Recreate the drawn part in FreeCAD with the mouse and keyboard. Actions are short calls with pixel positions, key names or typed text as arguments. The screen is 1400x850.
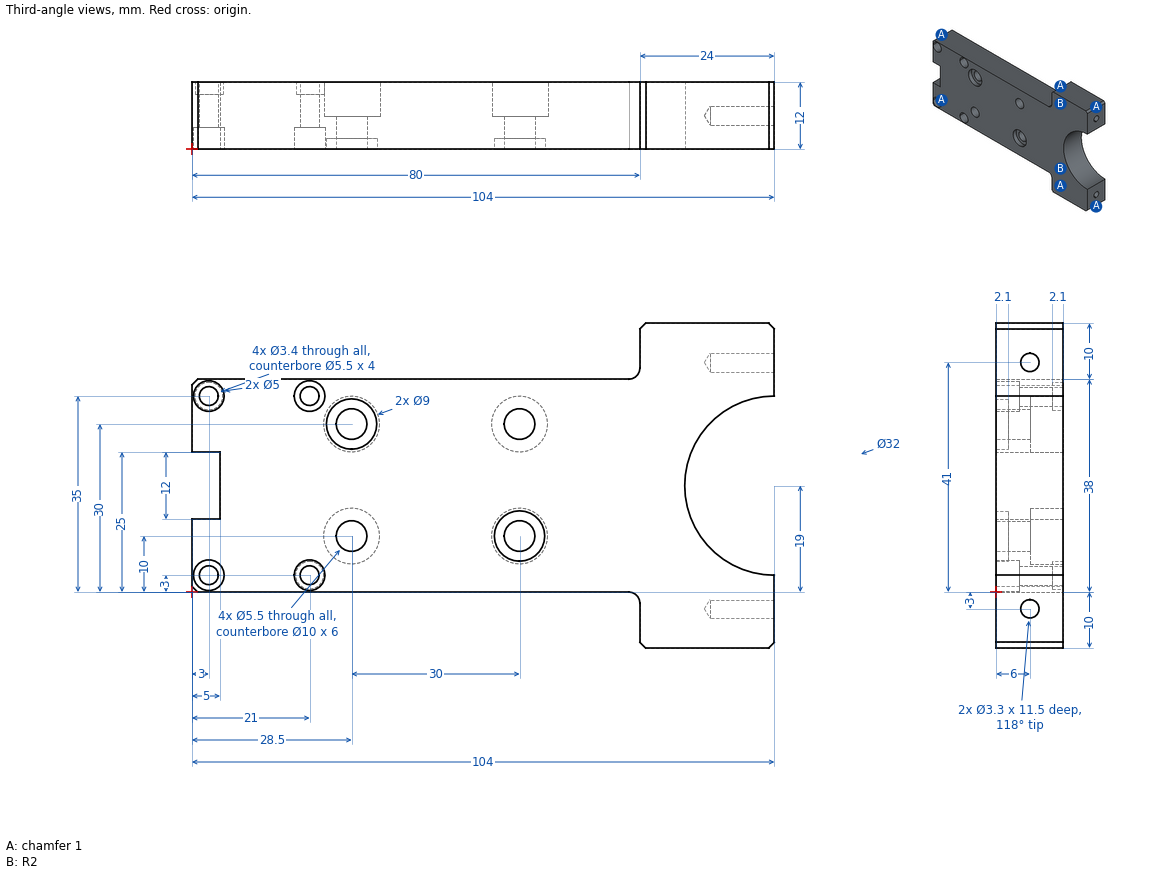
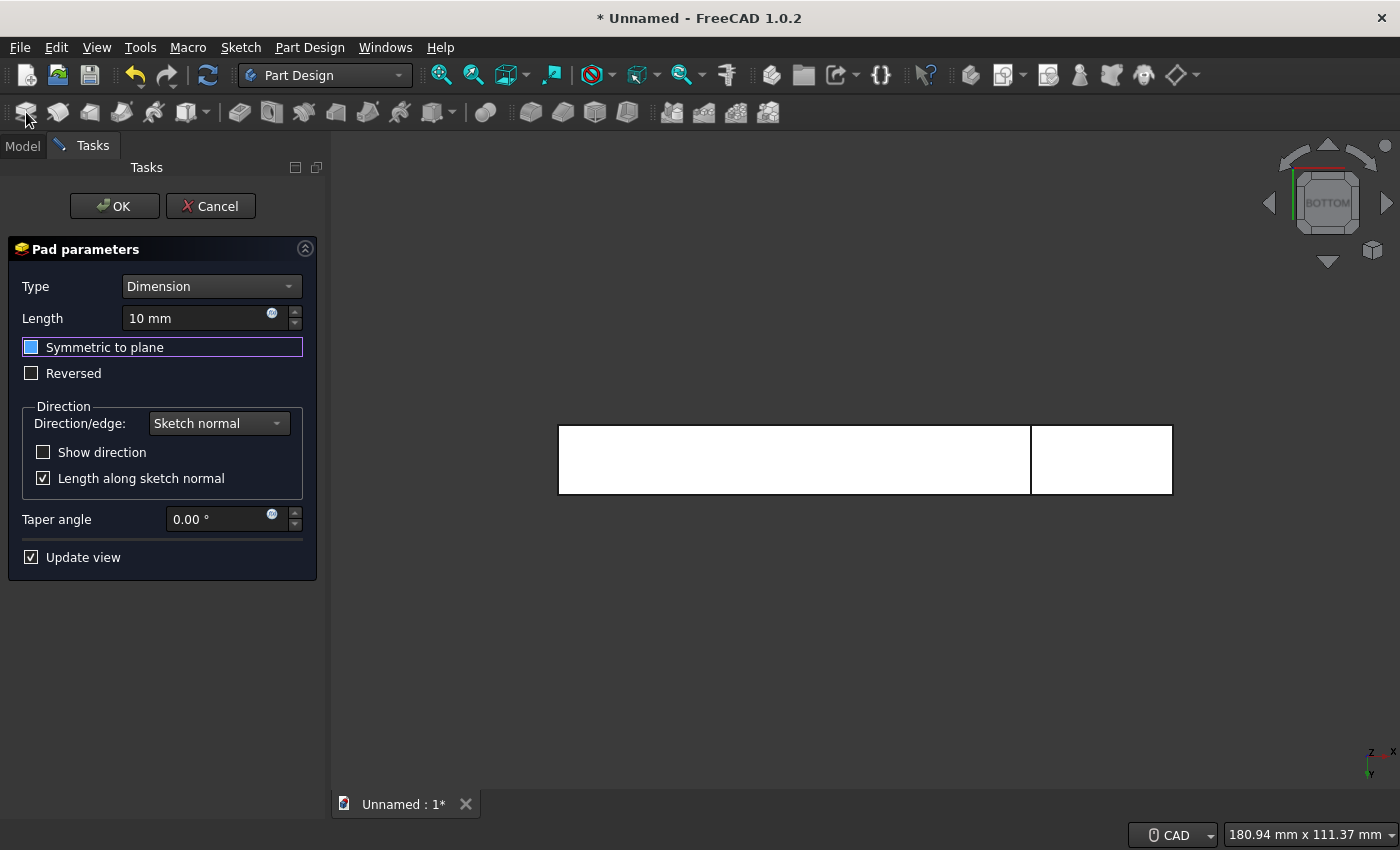
click(115, 206)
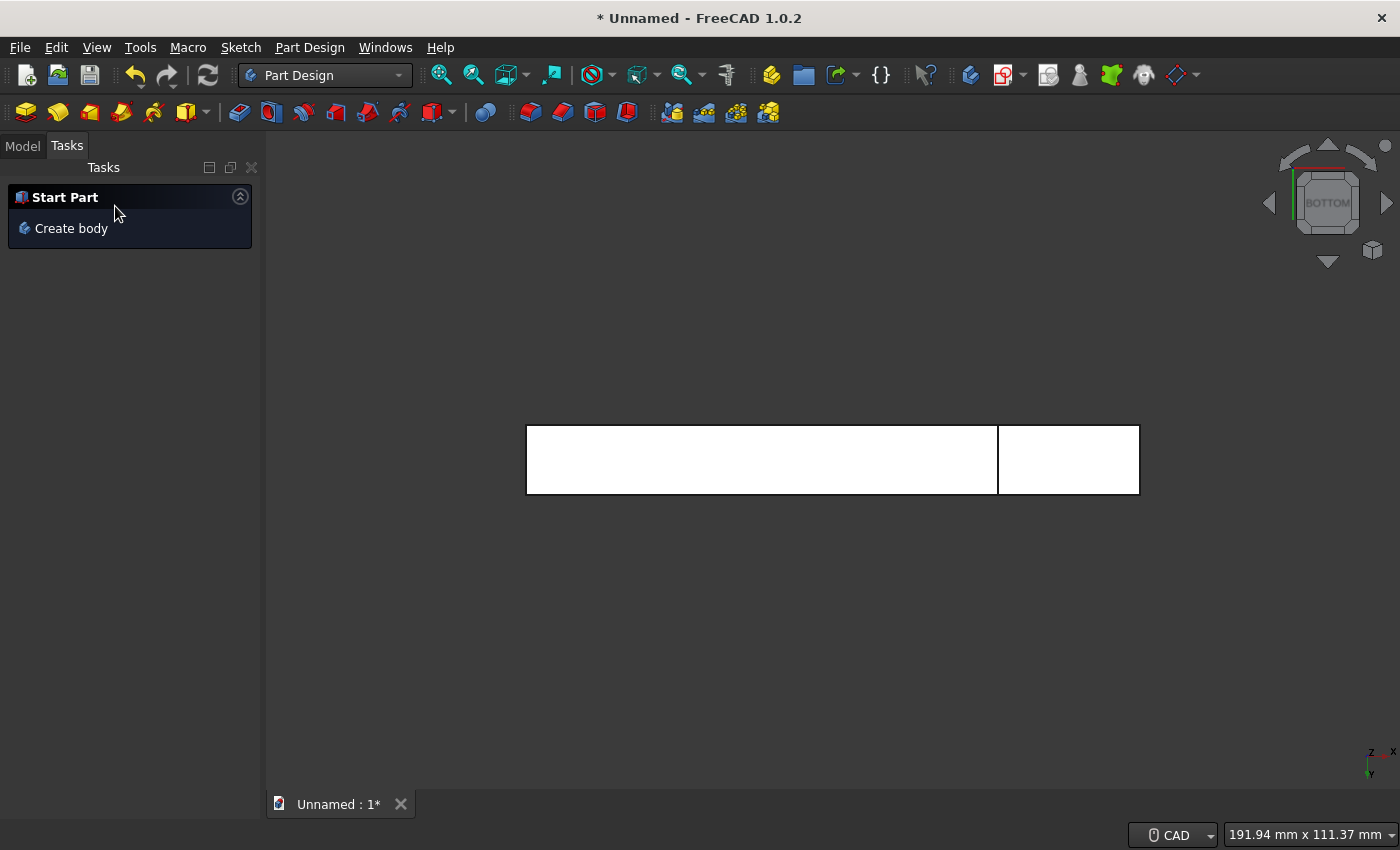
key(0)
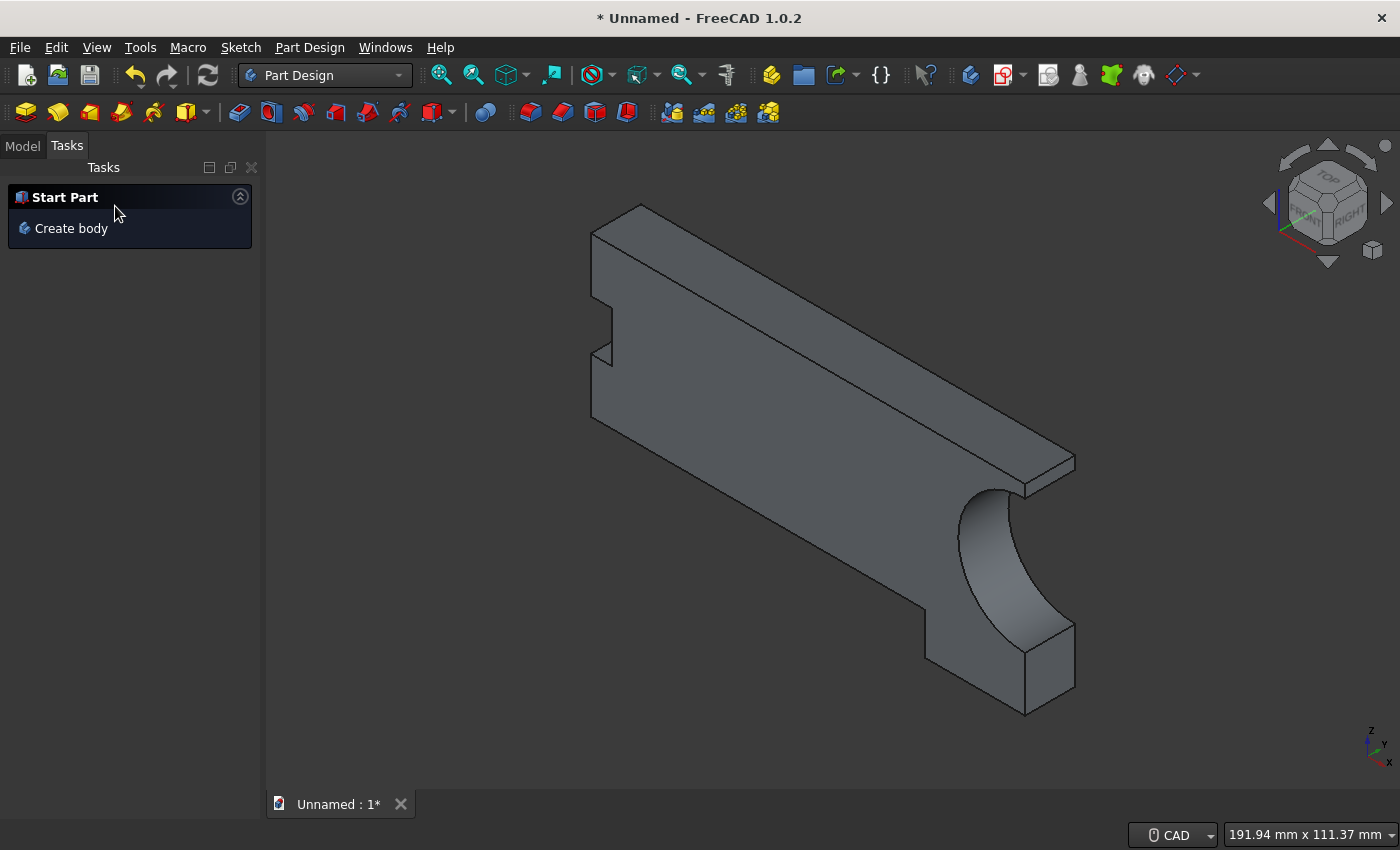
click(1019, 451)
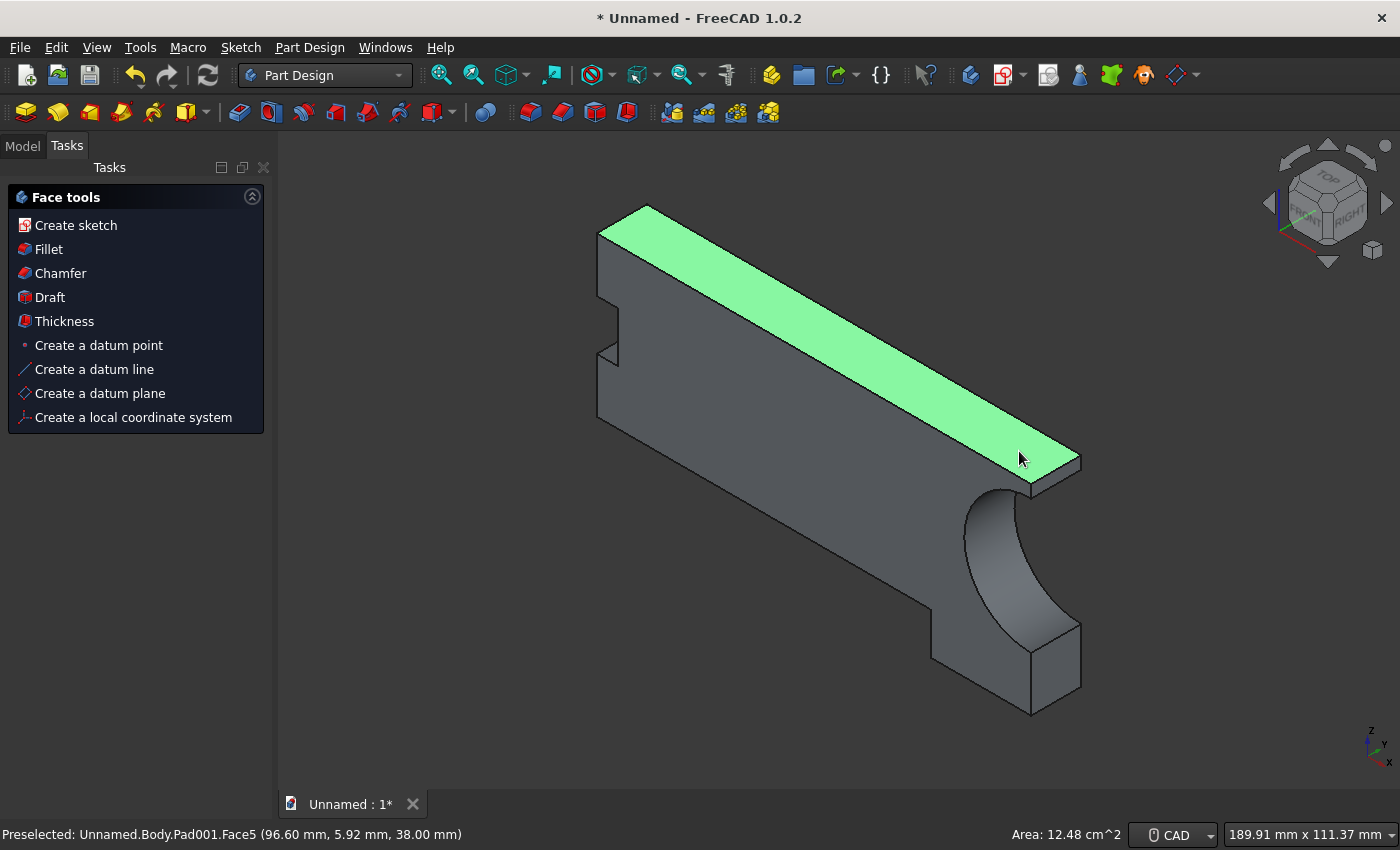
click(1004, 76)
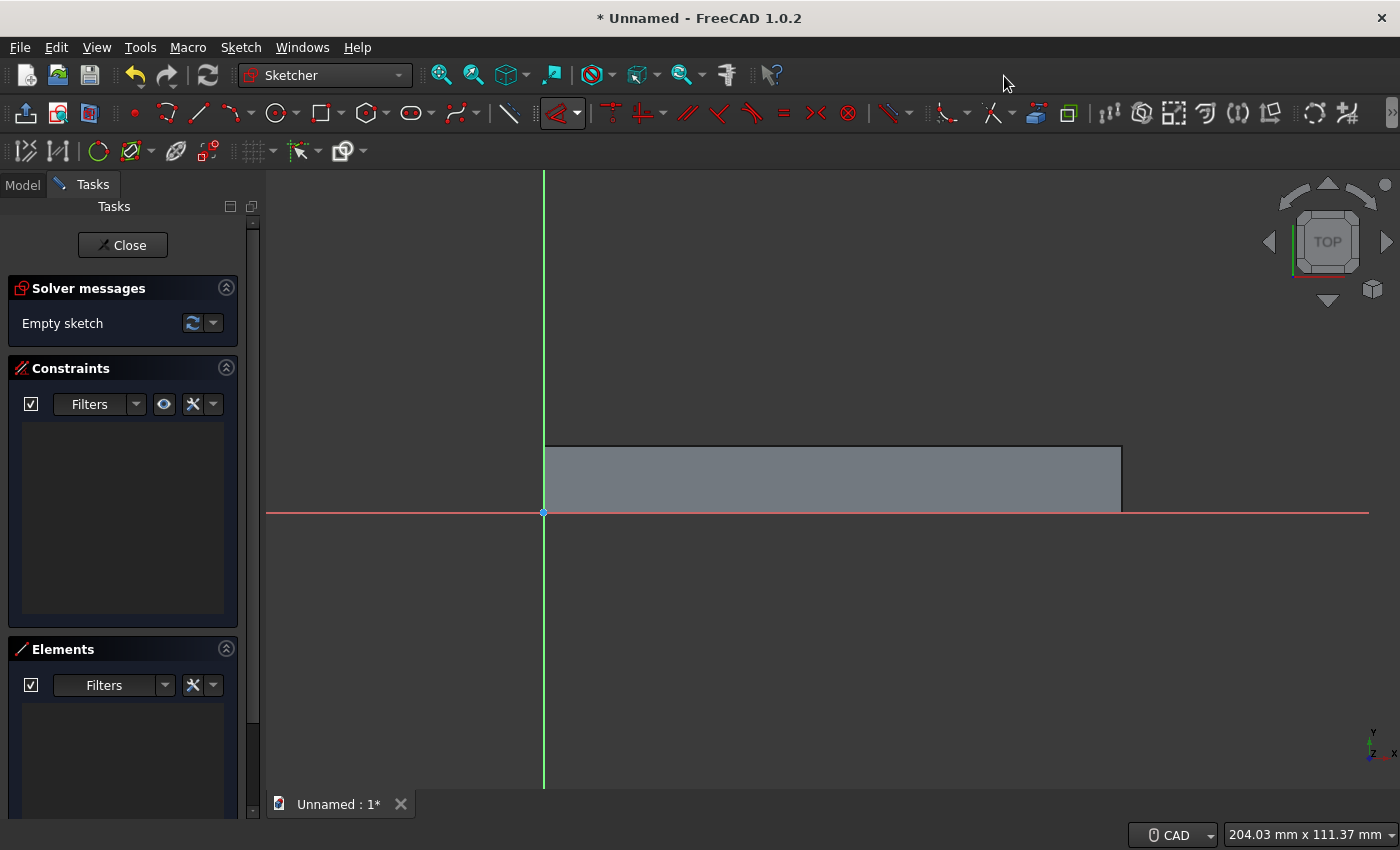
scroll(1129, 479, up, 8)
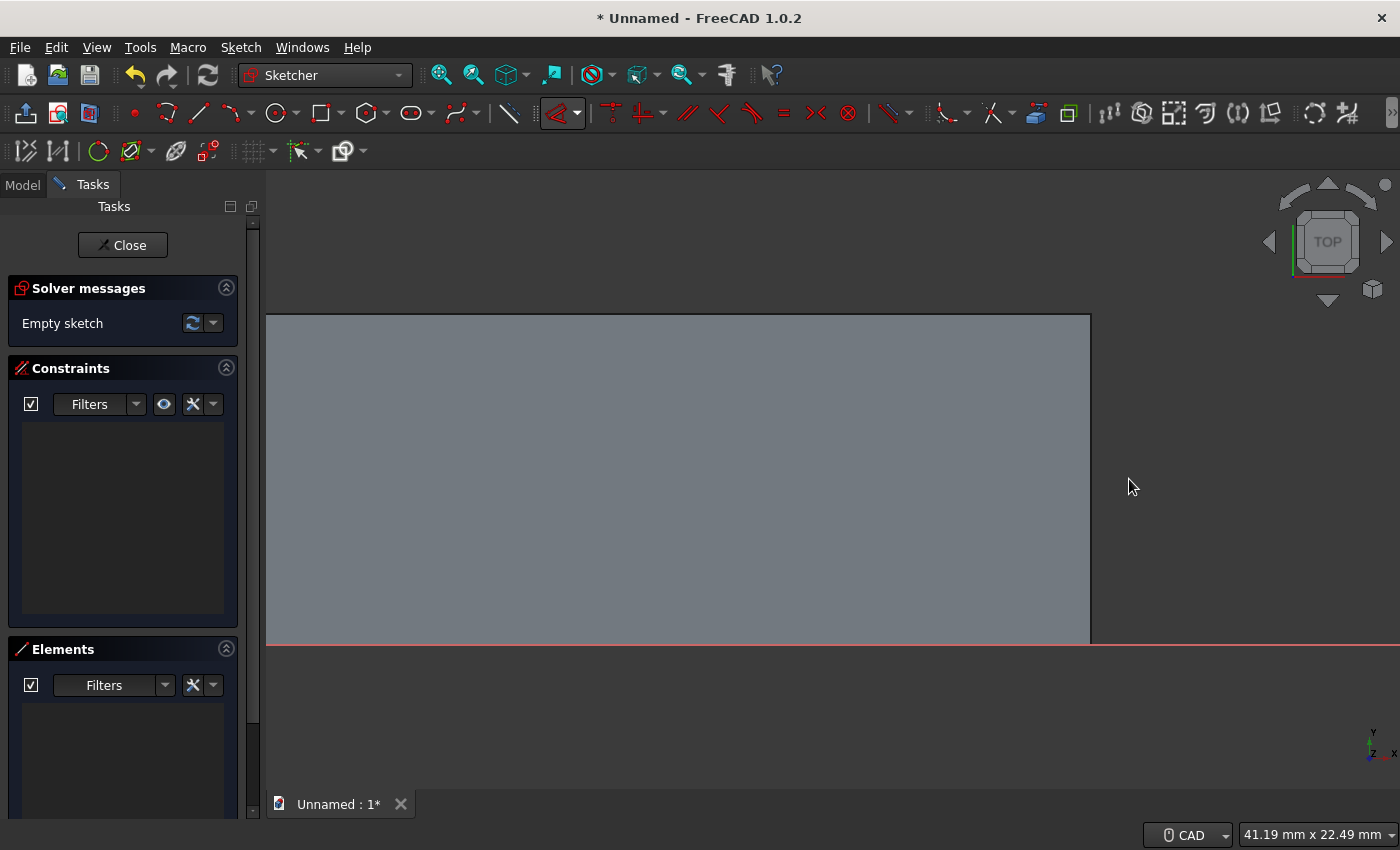
click(322, 114)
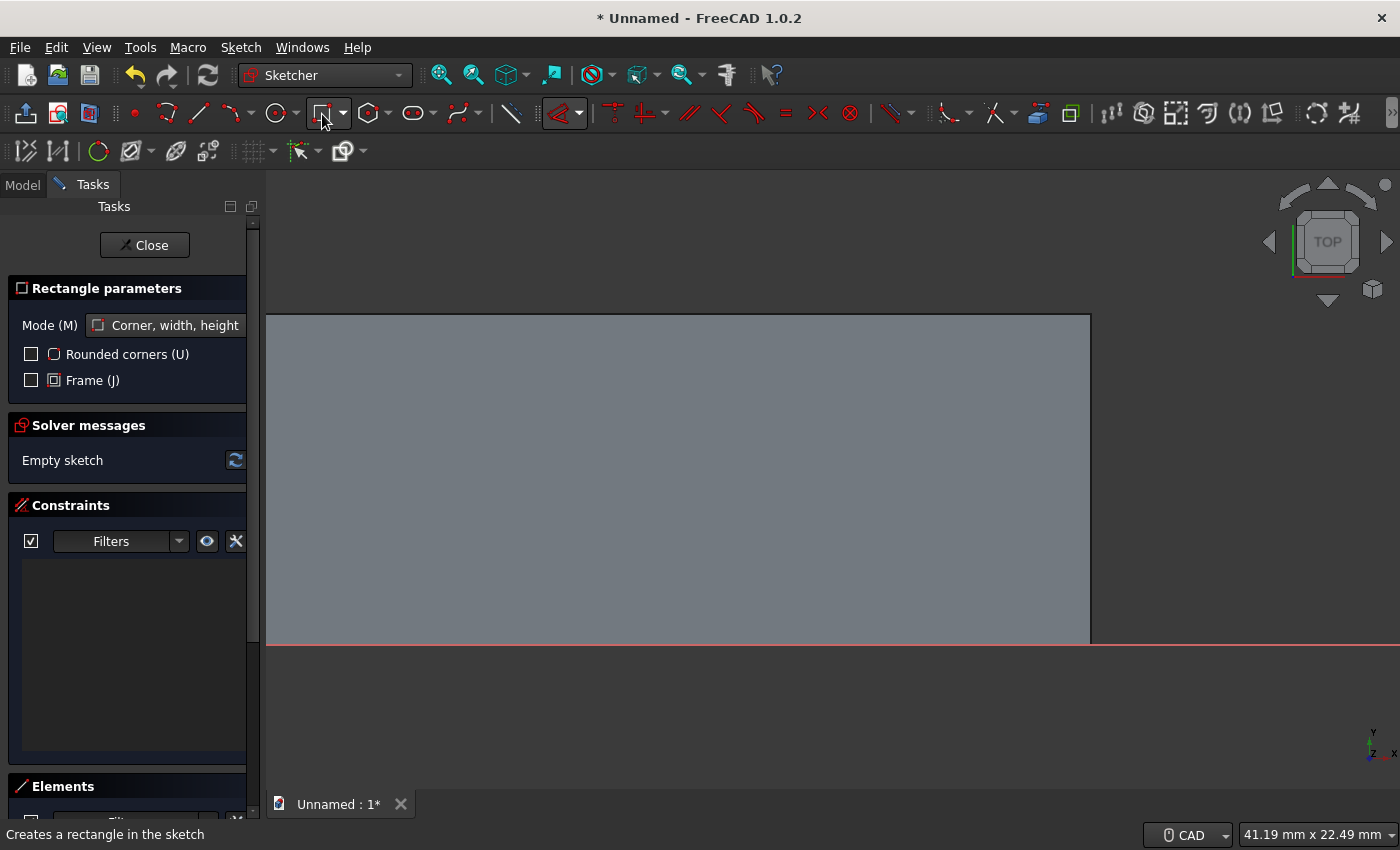
click(431, 314)
click(1091, 645)
key(Escape)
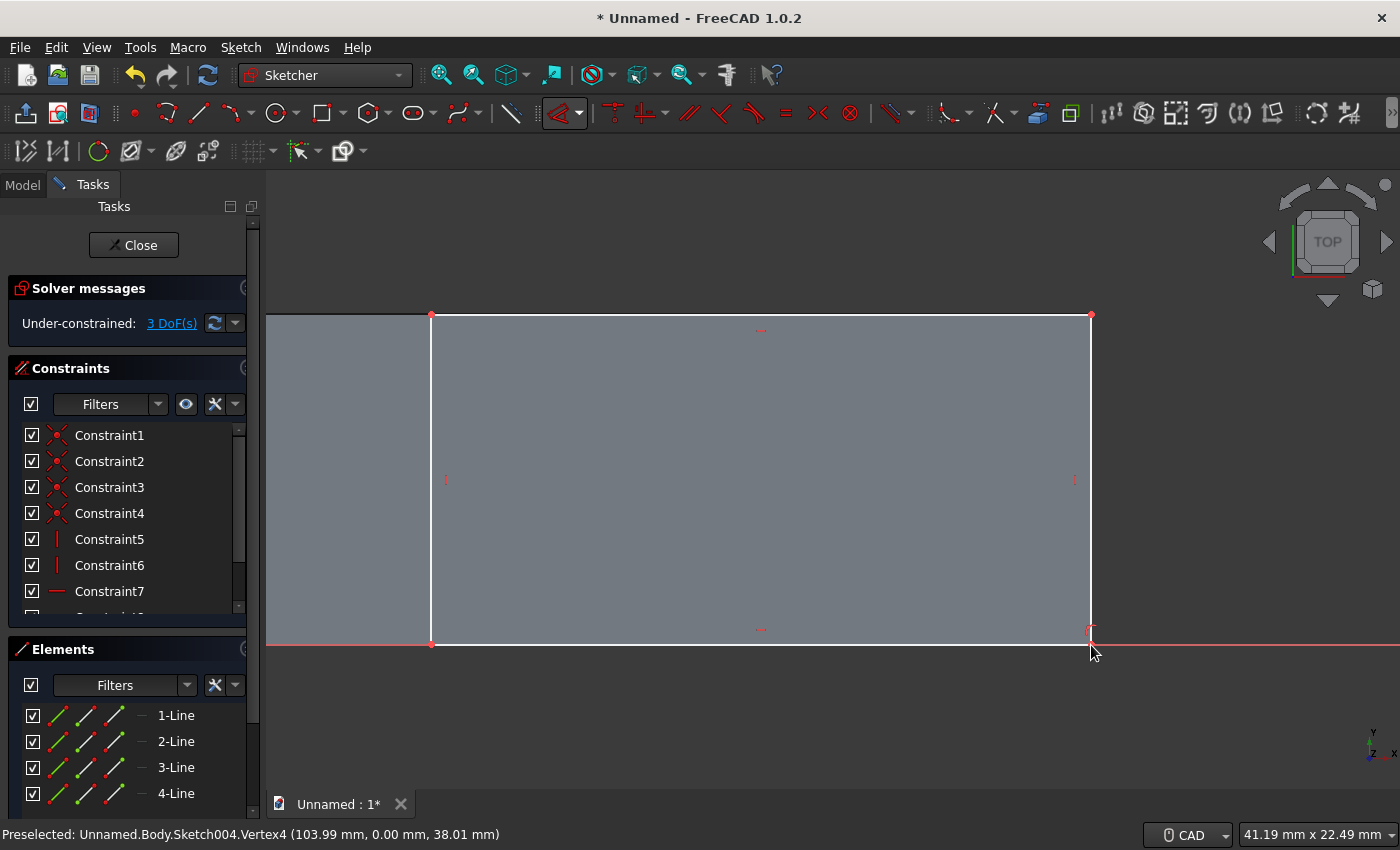
click(431, 414)